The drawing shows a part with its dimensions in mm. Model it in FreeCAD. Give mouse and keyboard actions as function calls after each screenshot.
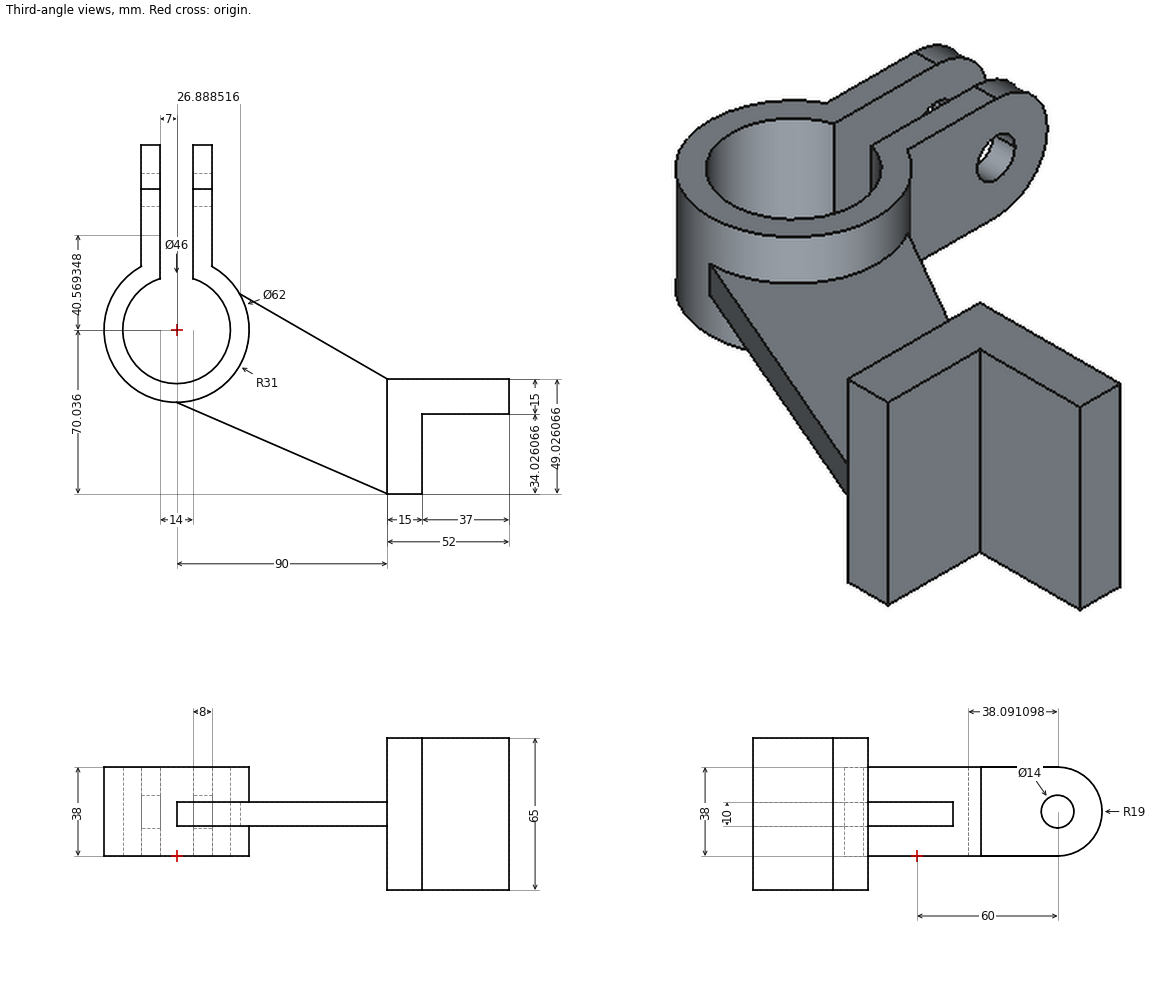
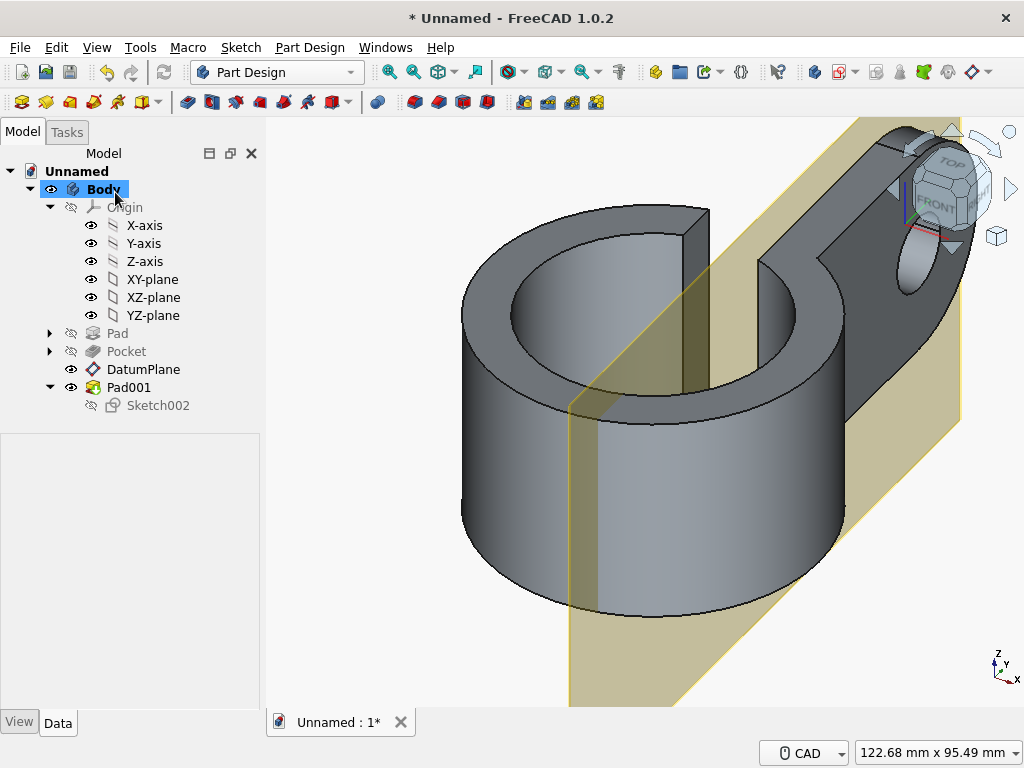
click(116, 369)
key(space)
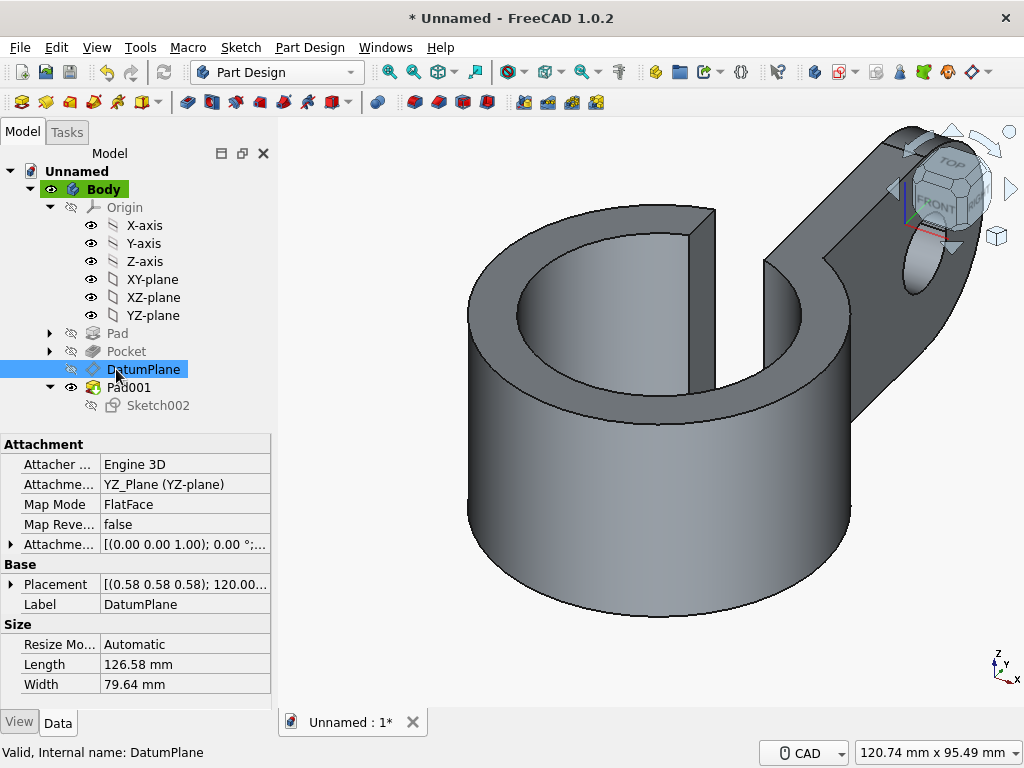
click(390, 72)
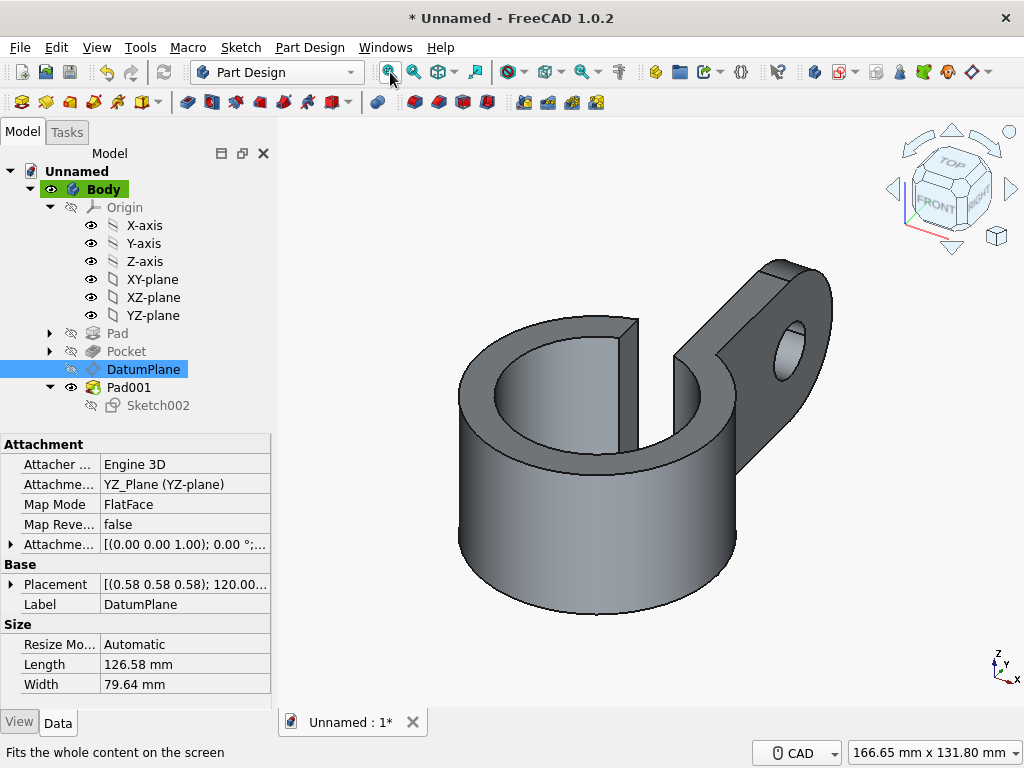
click(116, 387)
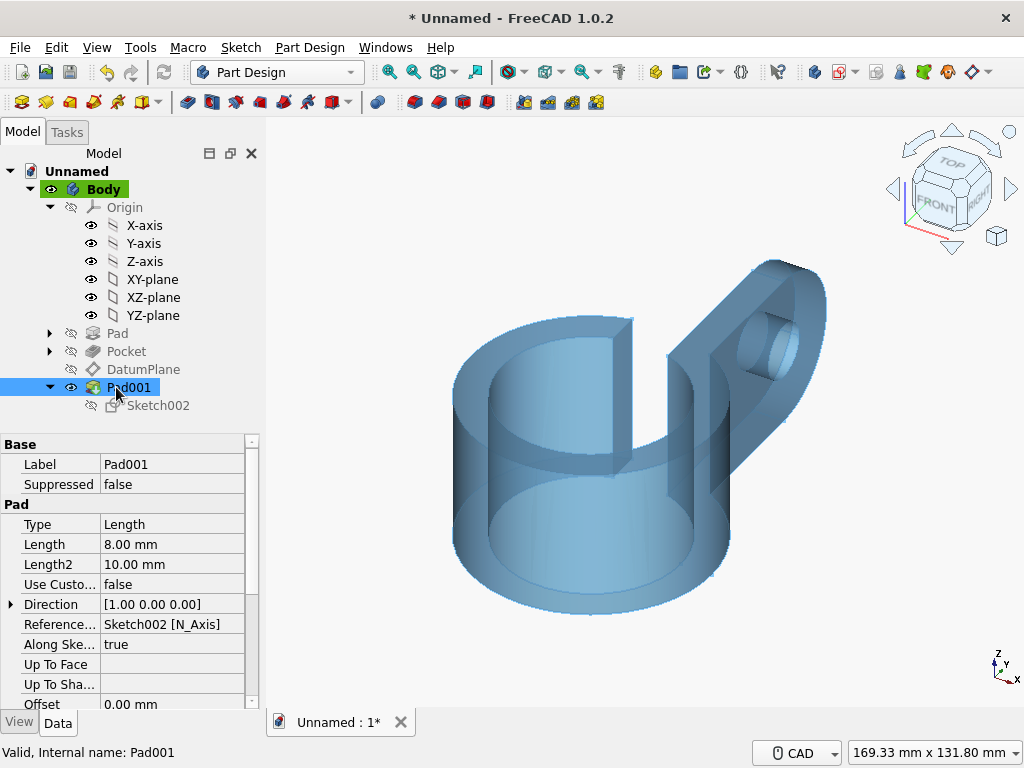
click(524, 102)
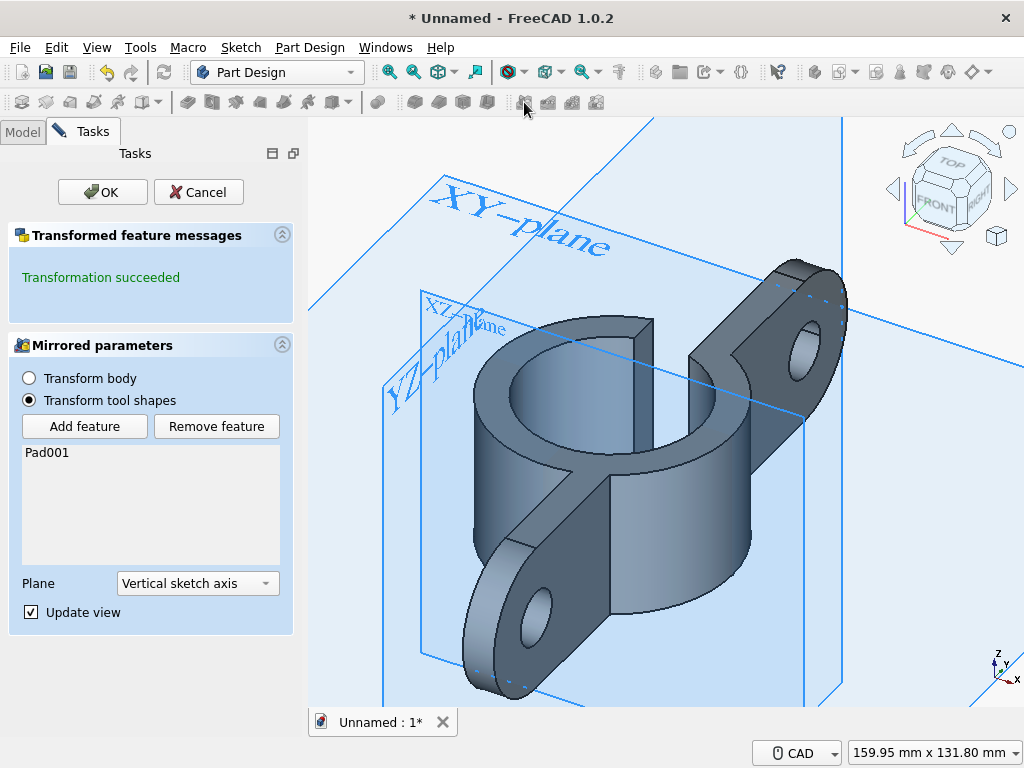
click(198, 584)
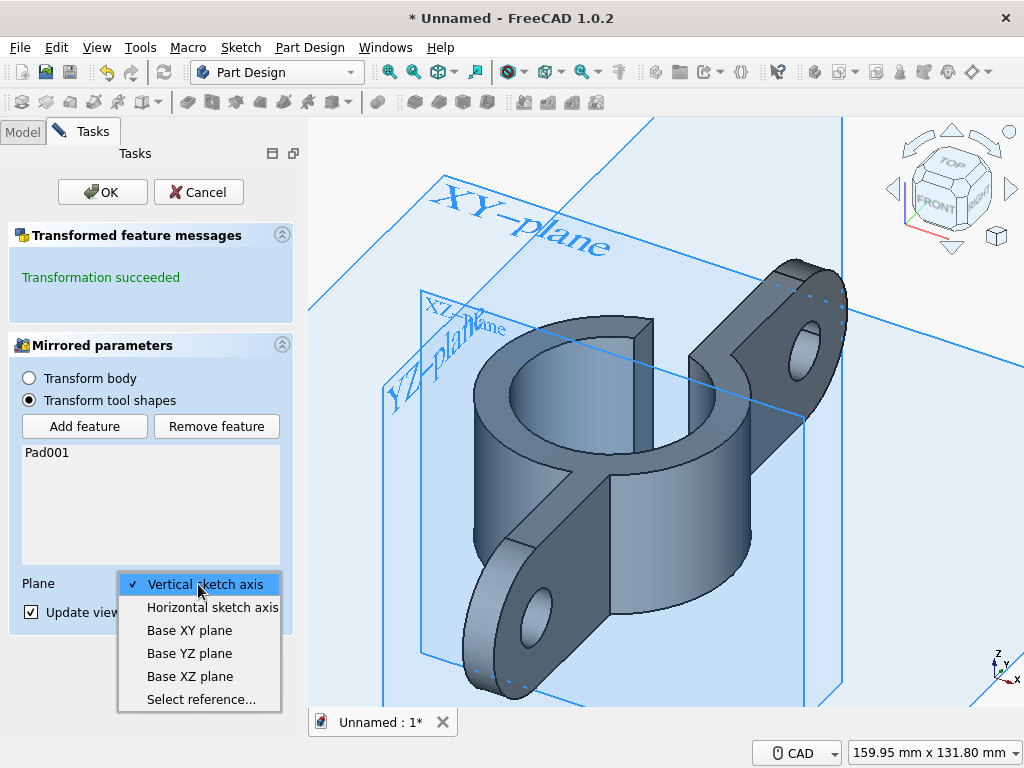
click(198, 654)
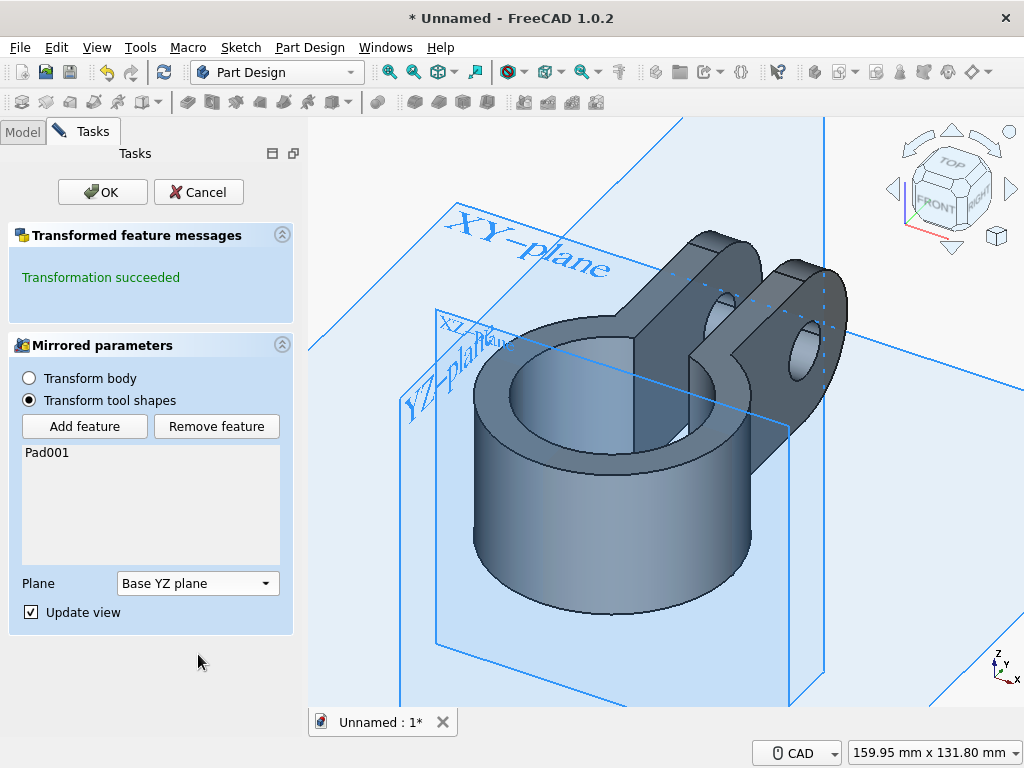
click(103, 192)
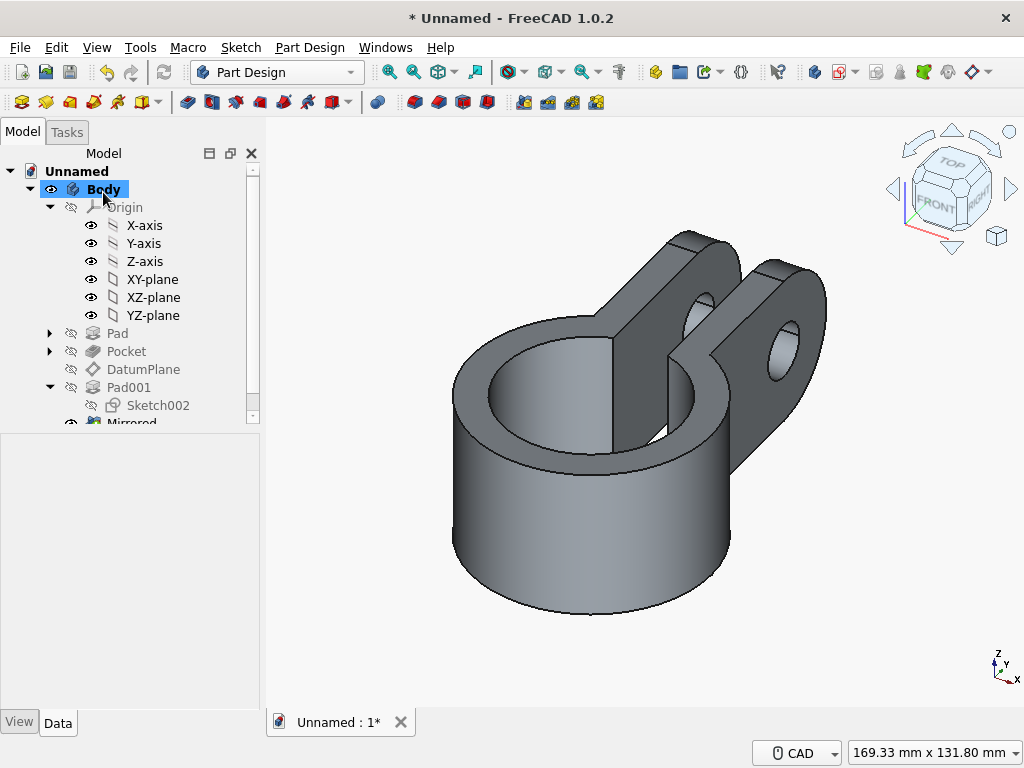
click(816, 72)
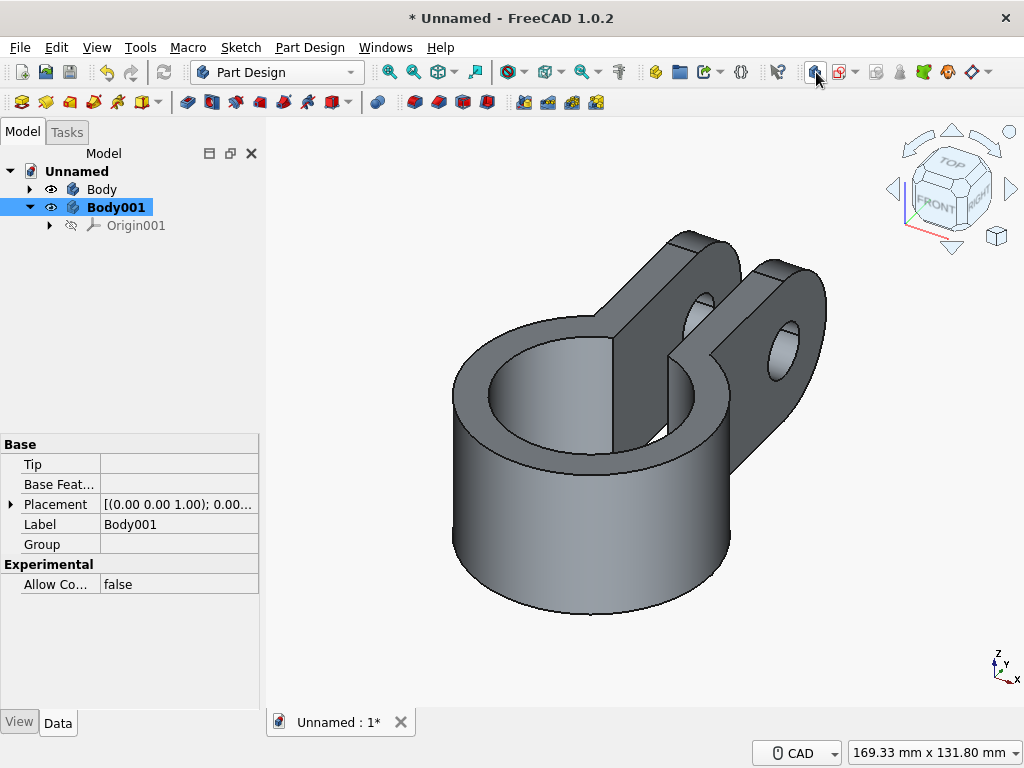
click(50, 225)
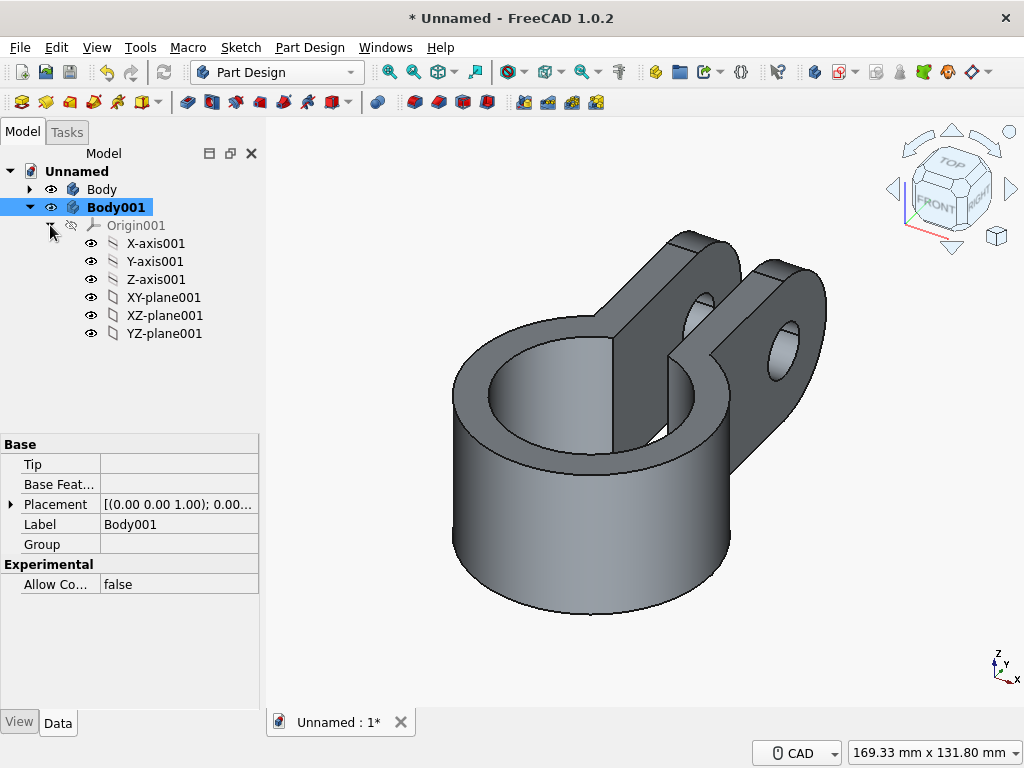
click(136, 297)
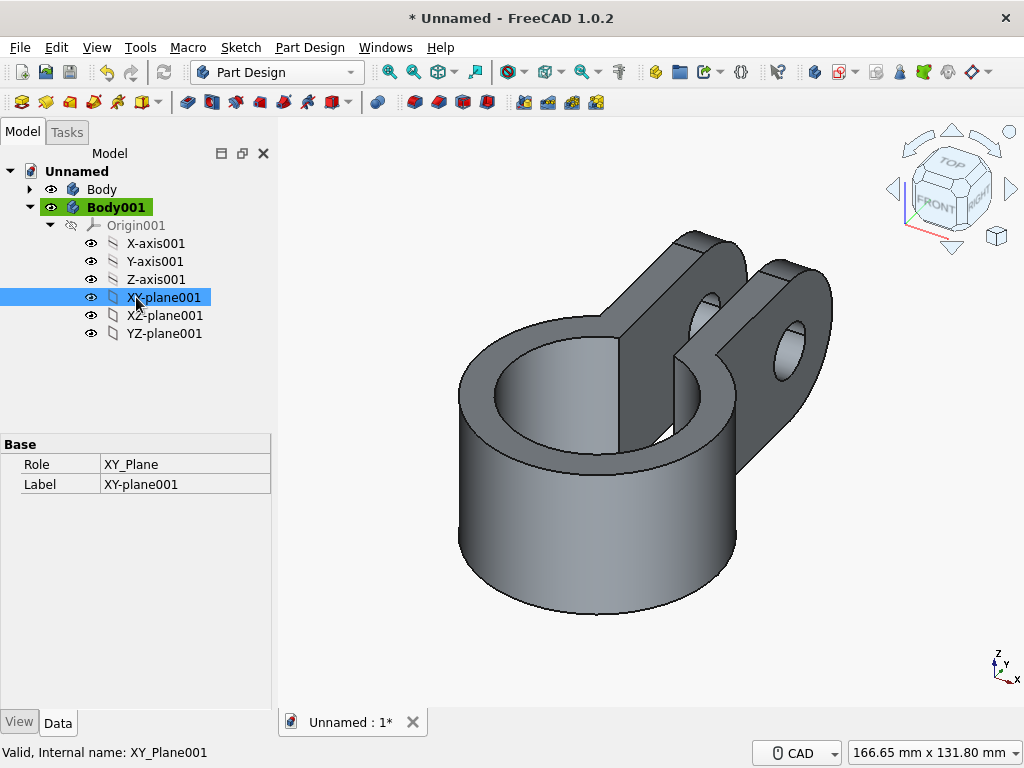
click(972, 72)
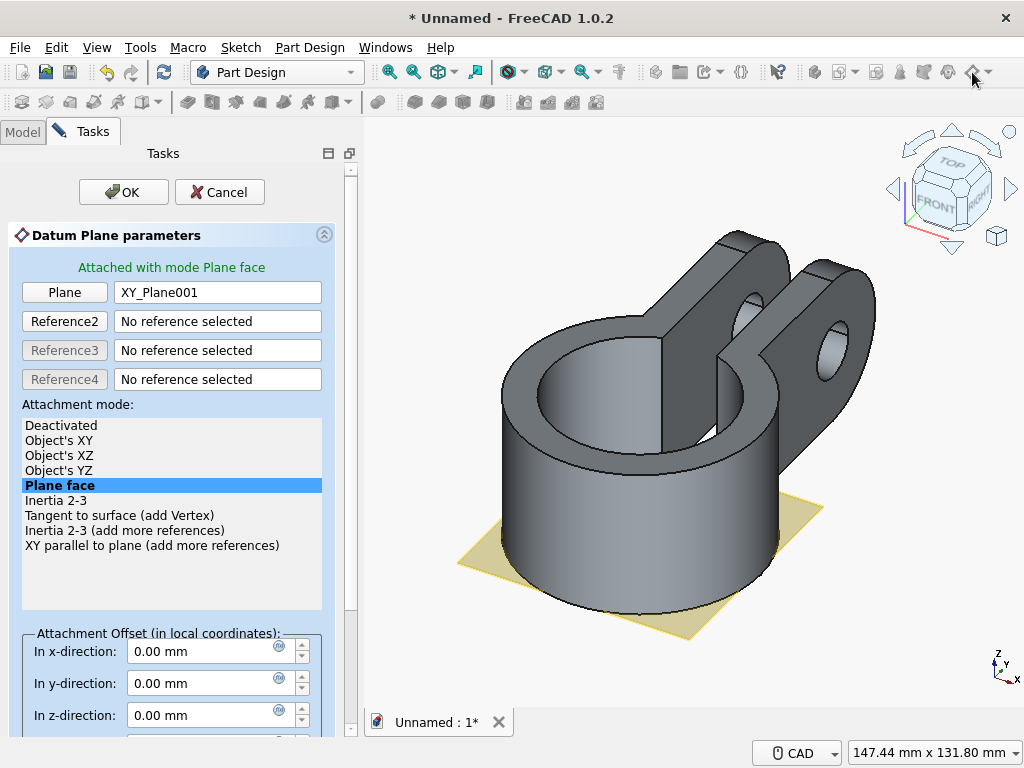
triple_click(210, 715)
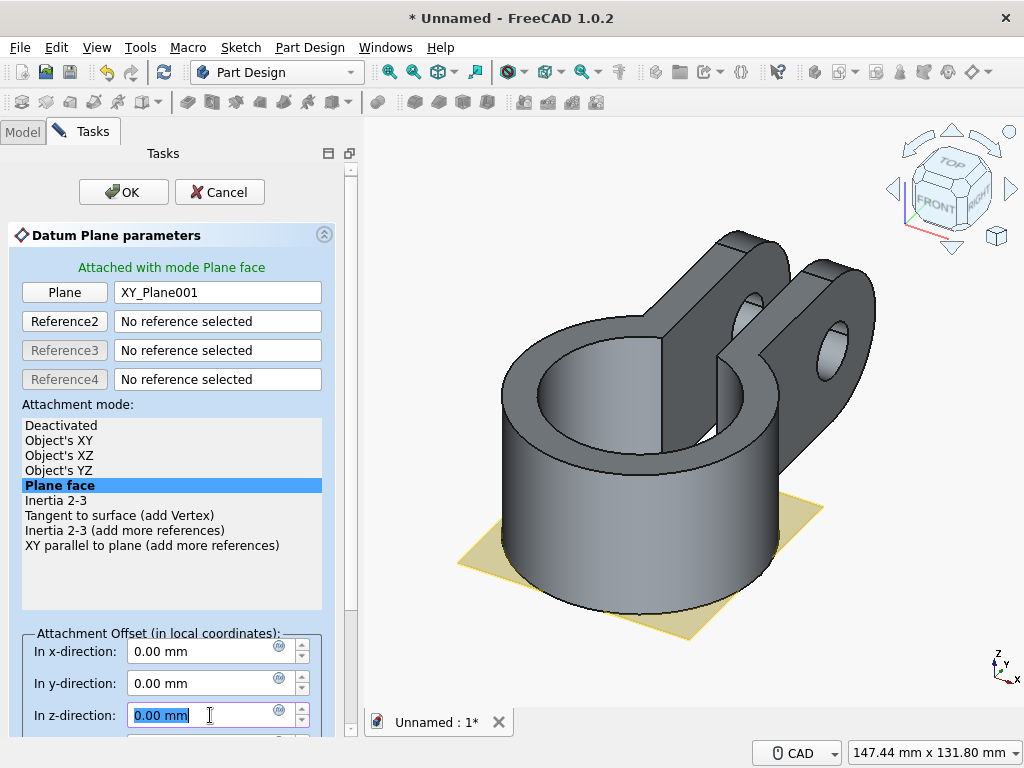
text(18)
key(Tab)